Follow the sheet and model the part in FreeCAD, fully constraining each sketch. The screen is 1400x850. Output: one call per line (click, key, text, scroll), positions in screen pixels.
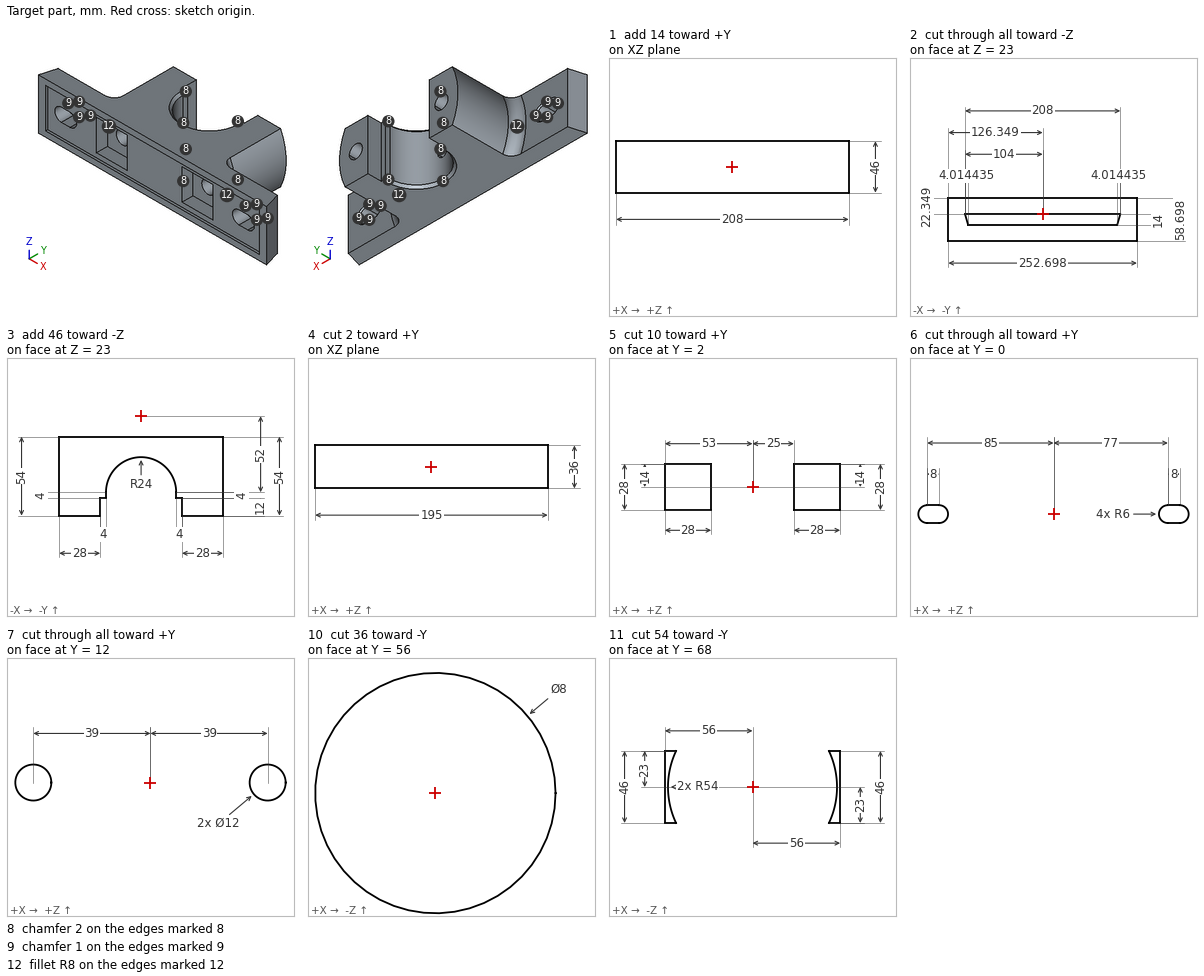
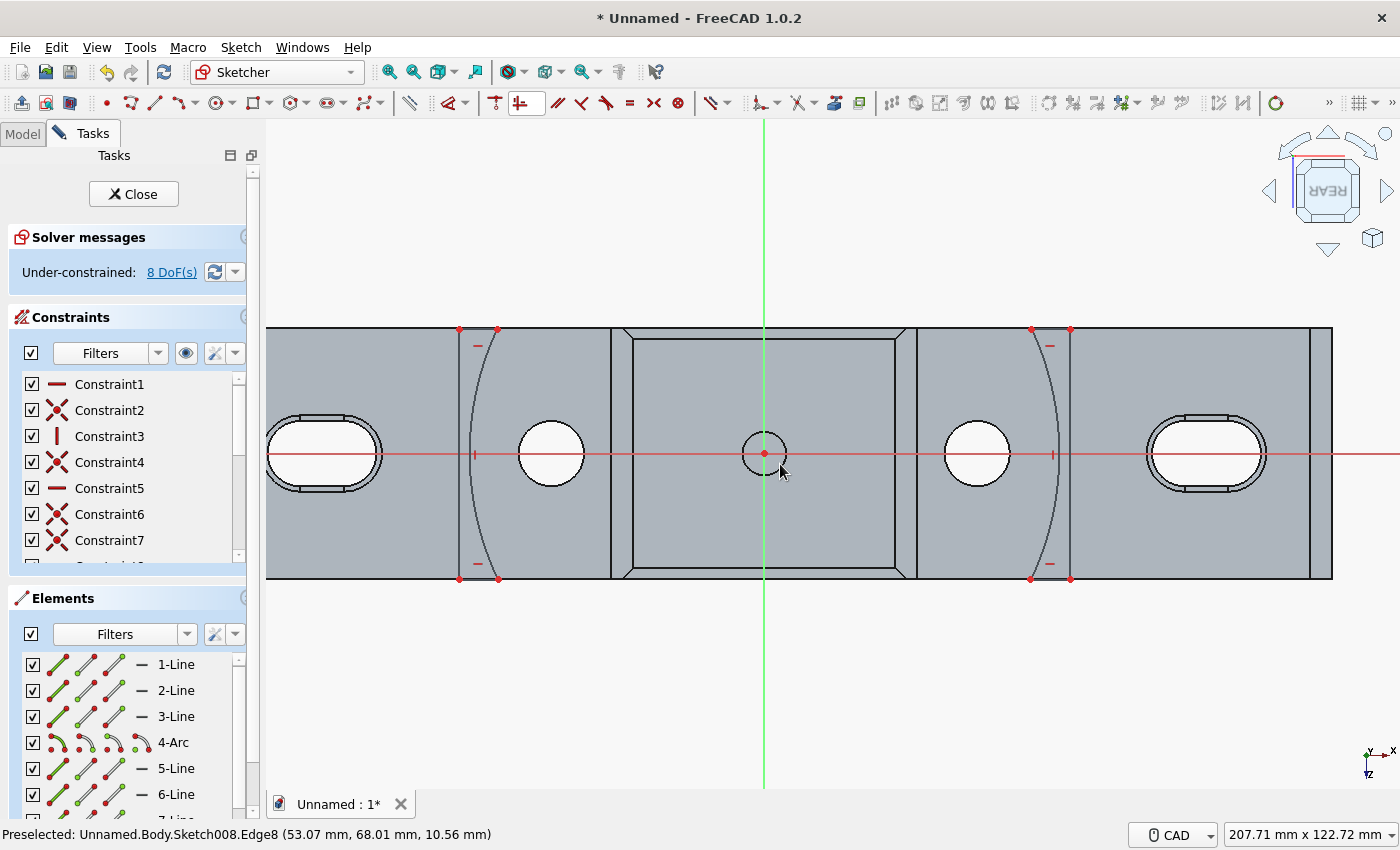
click(474, 403)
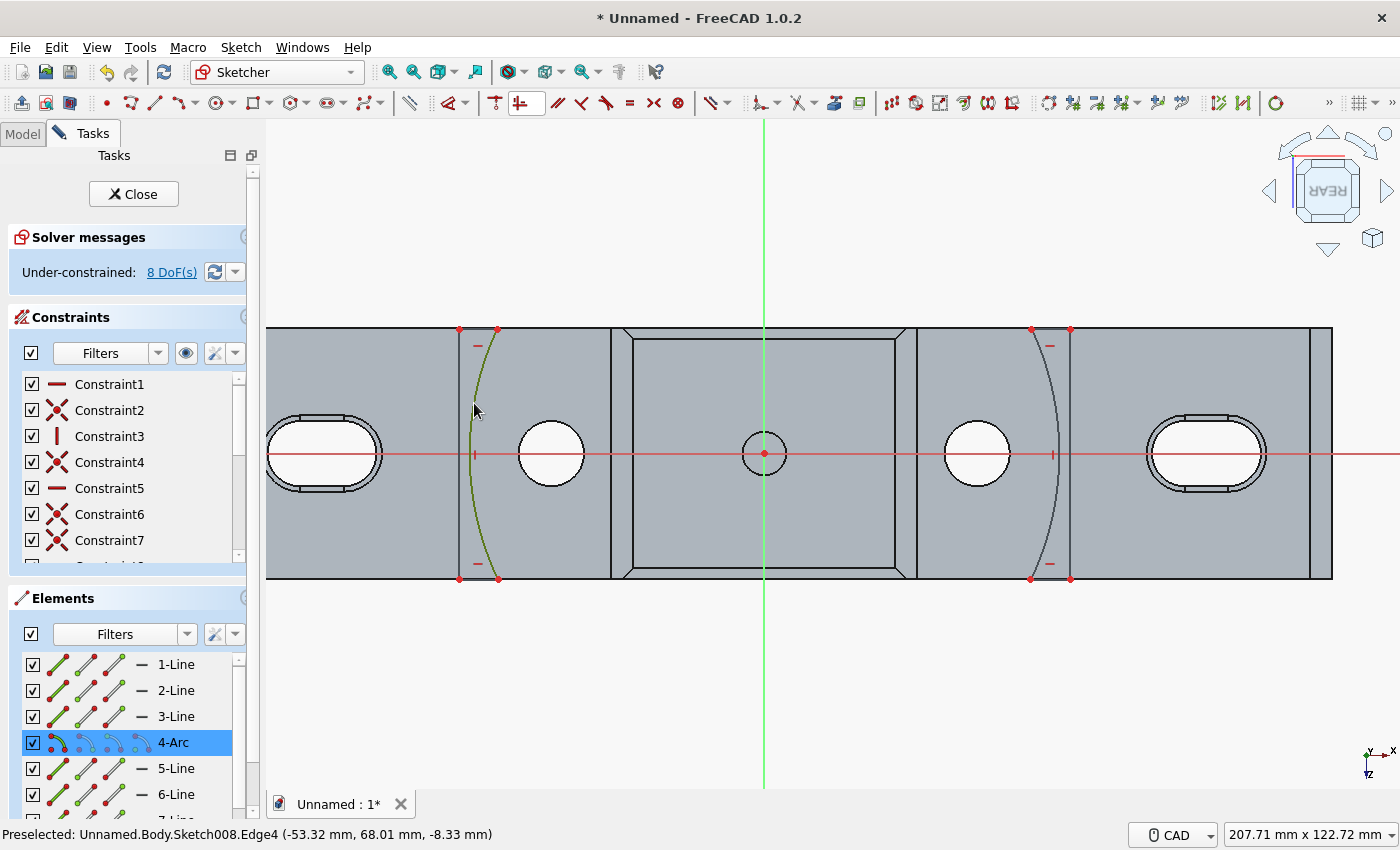
click(1055, 506)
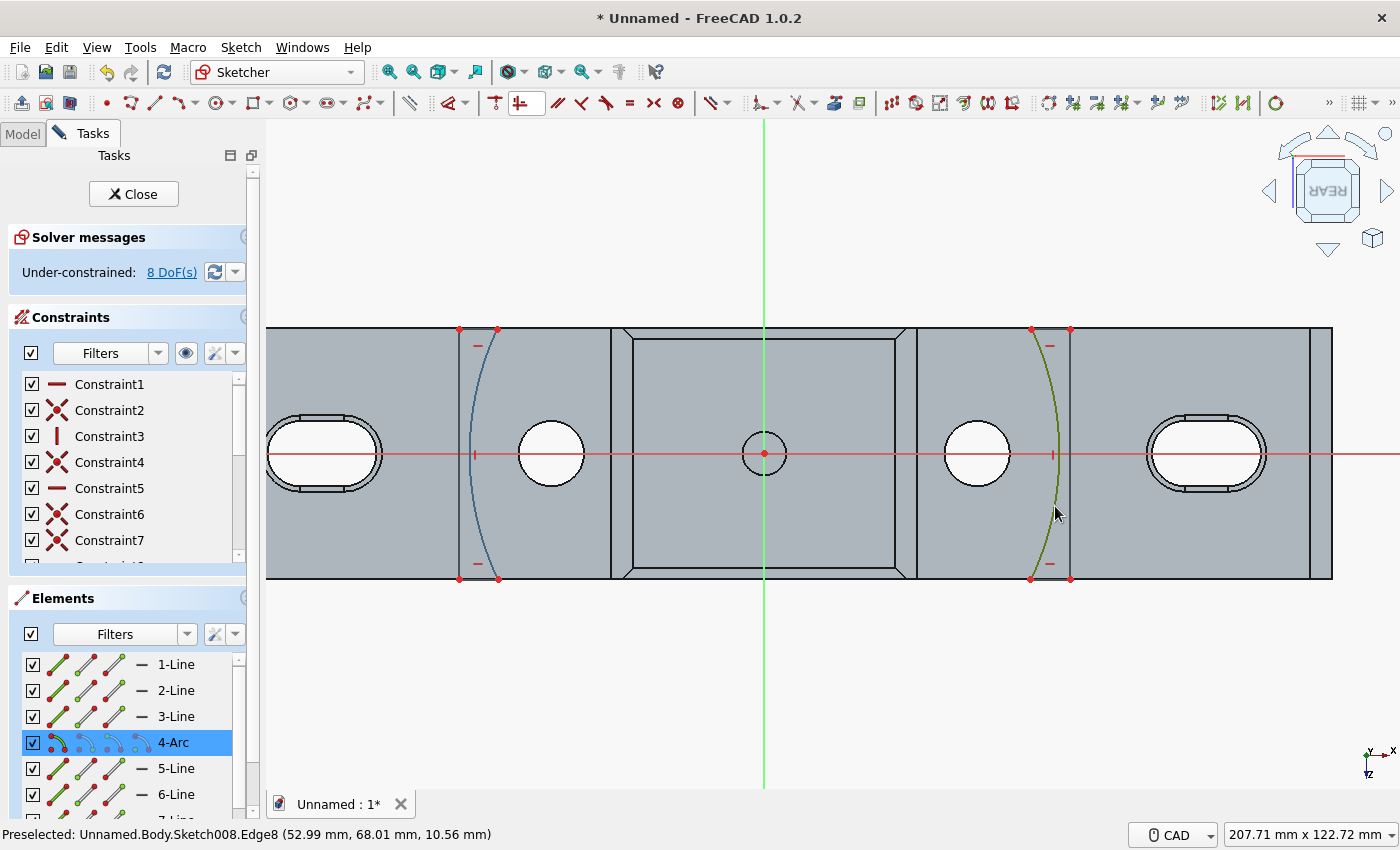
key(e)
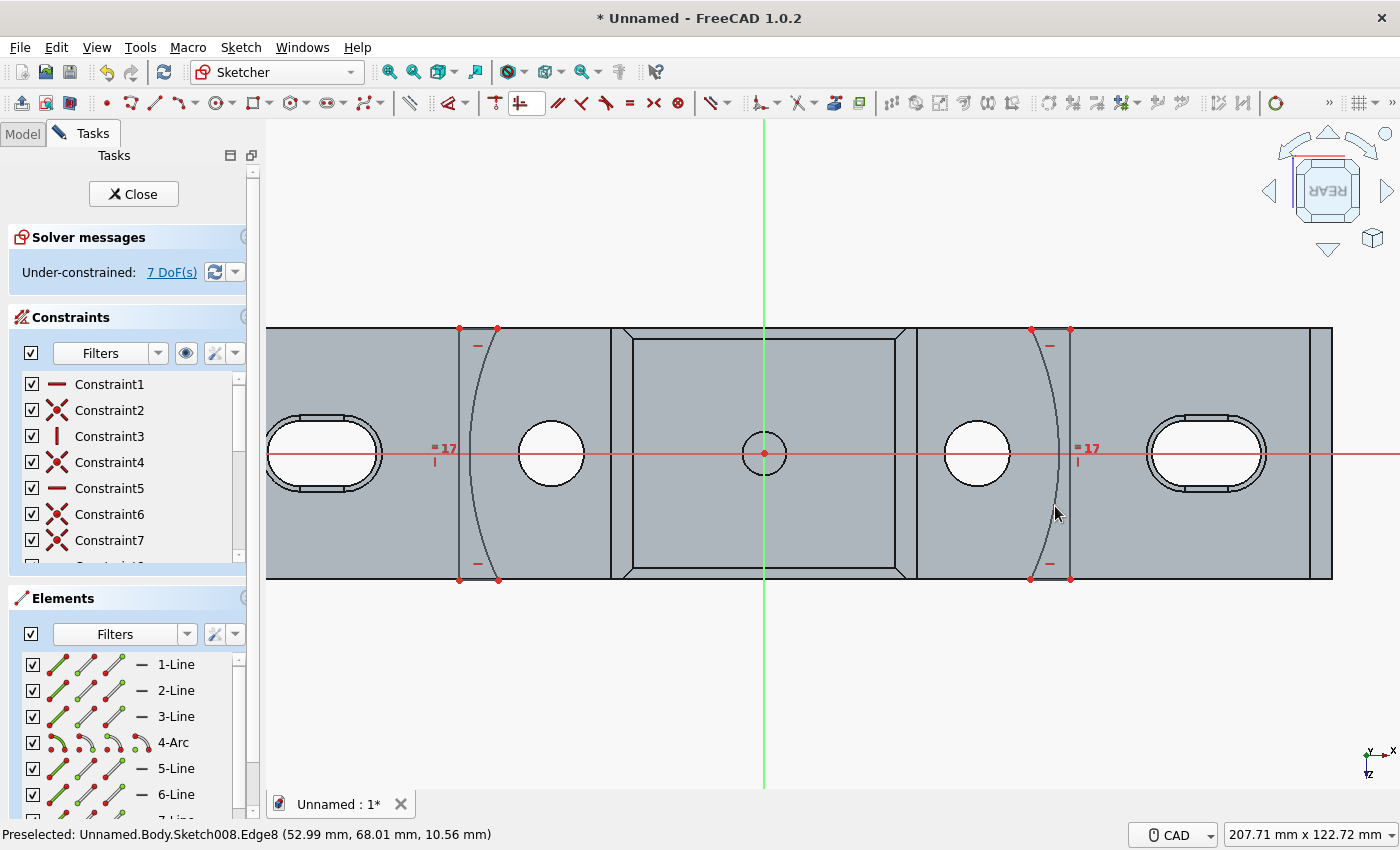
key(d)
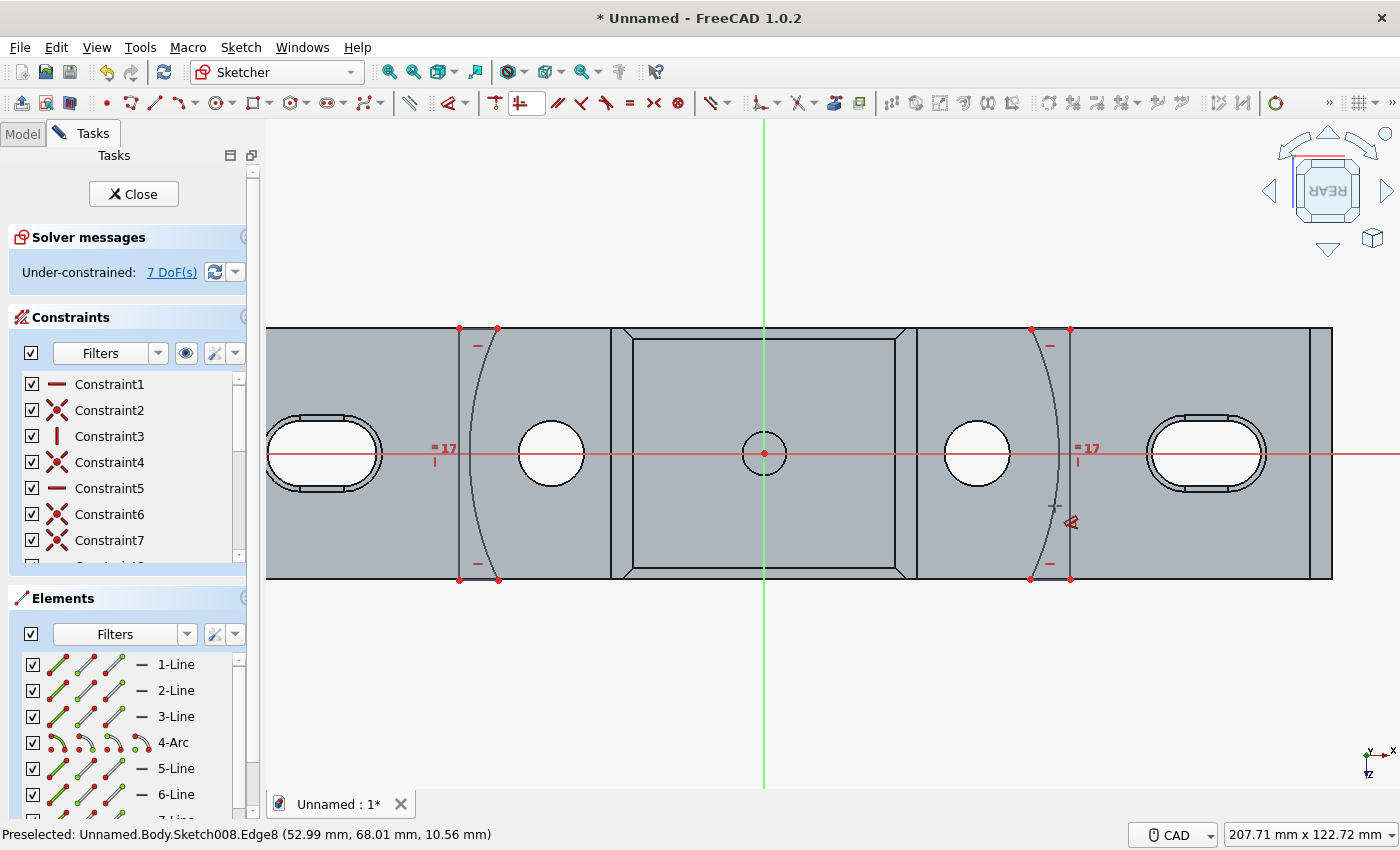
click(474, 403)
click(442, 398)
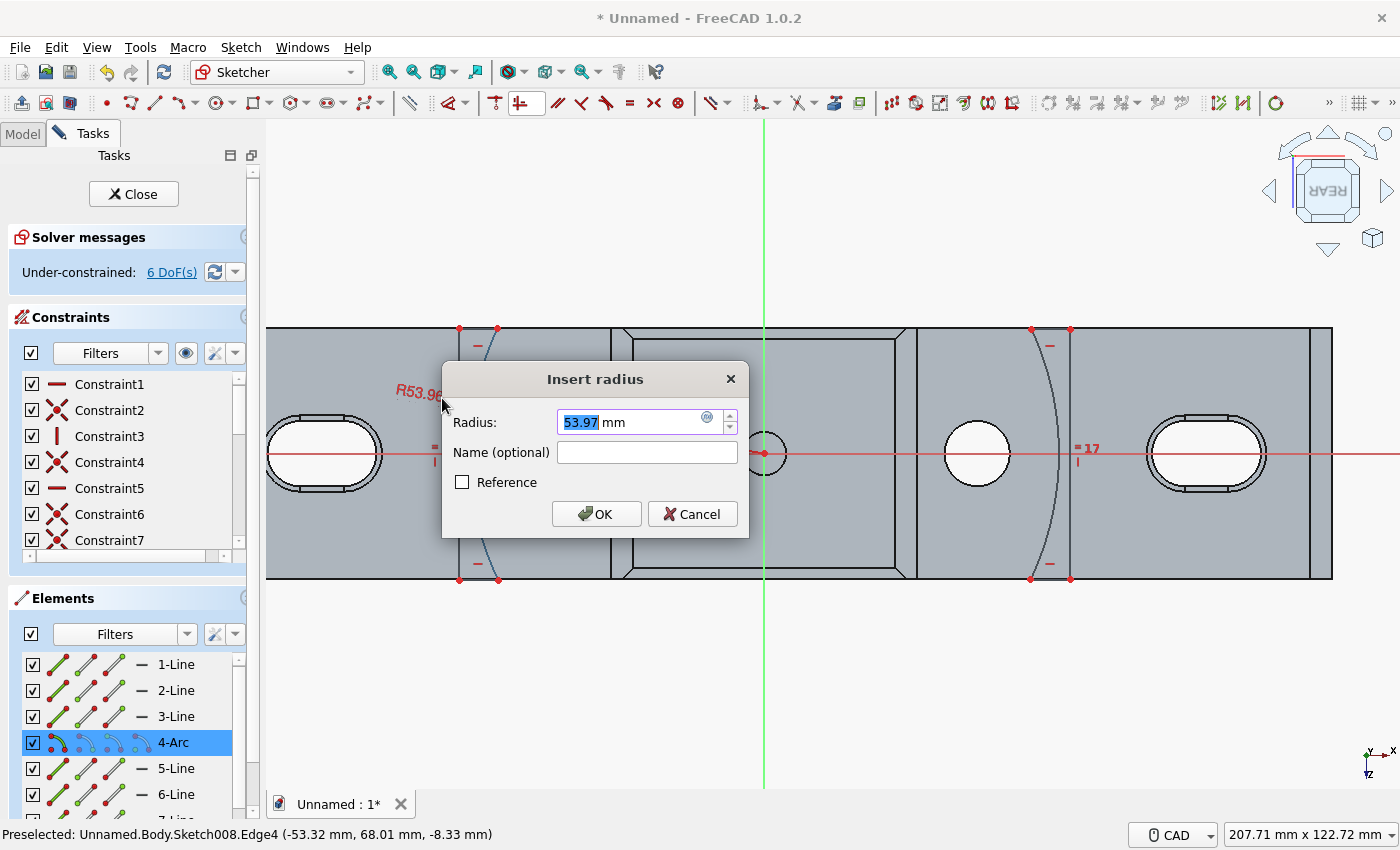
text(54)
key(Return)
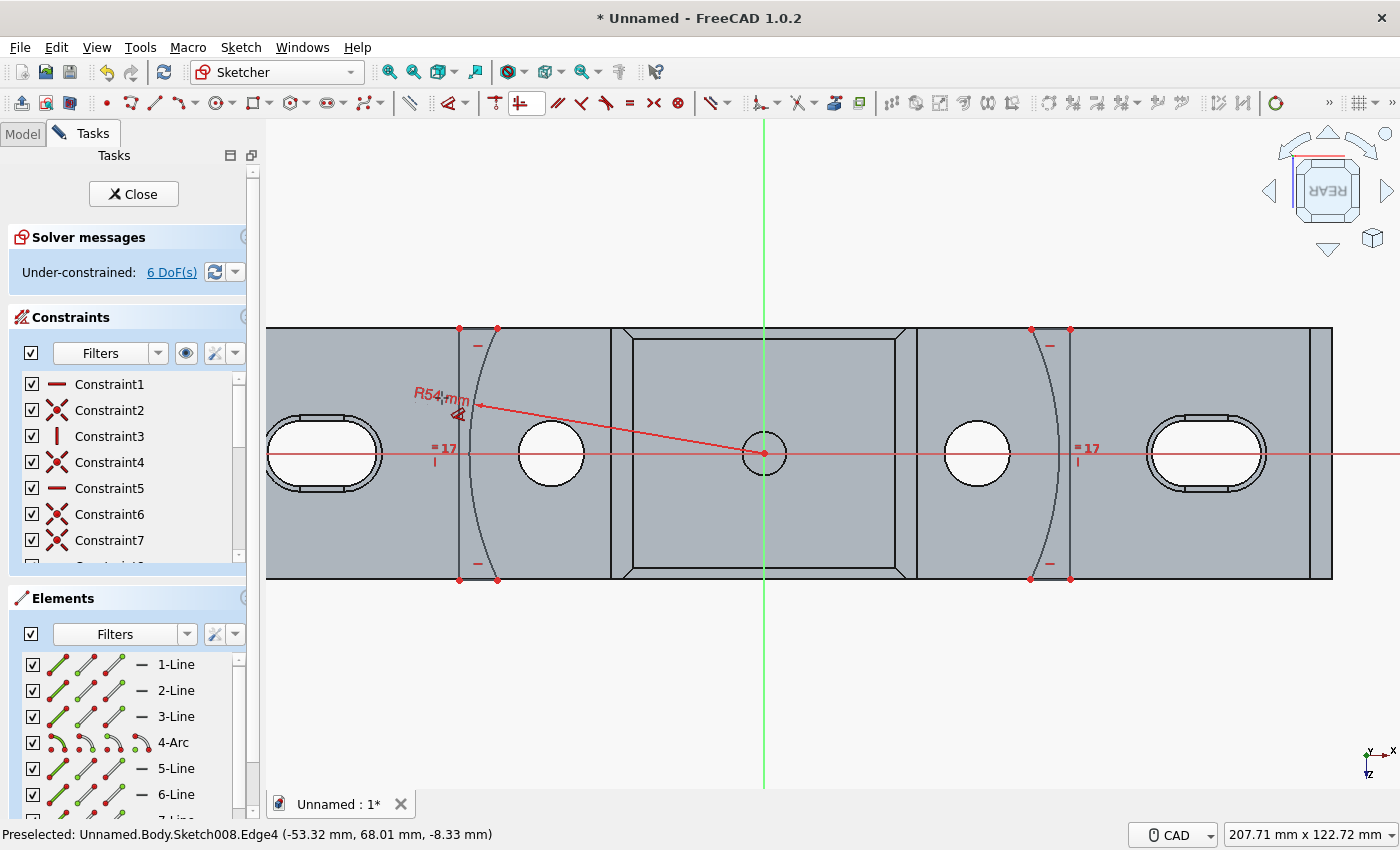
click(459, 404)
click(425, 512)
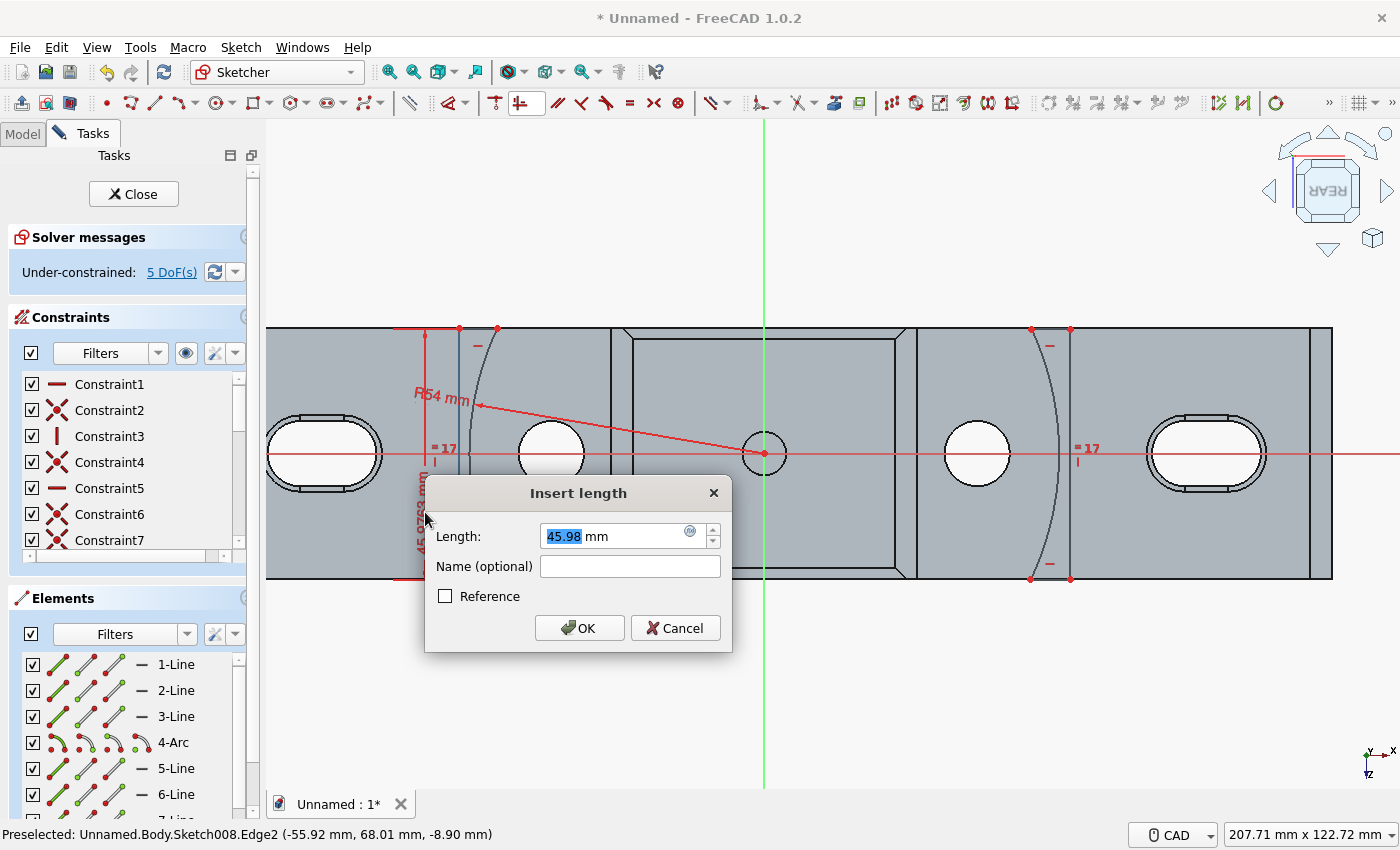
text(46)
key(Return)